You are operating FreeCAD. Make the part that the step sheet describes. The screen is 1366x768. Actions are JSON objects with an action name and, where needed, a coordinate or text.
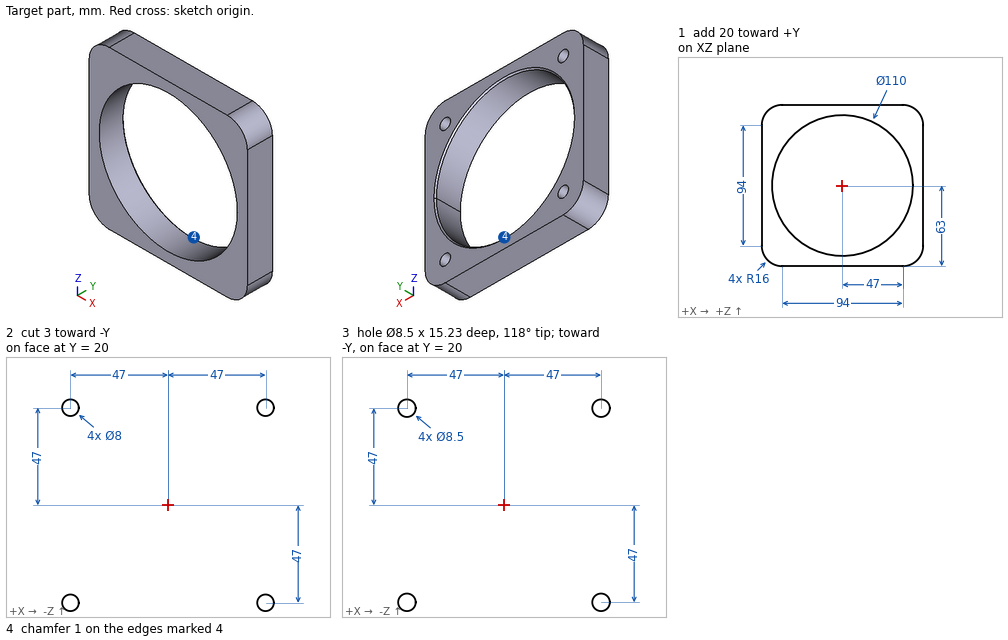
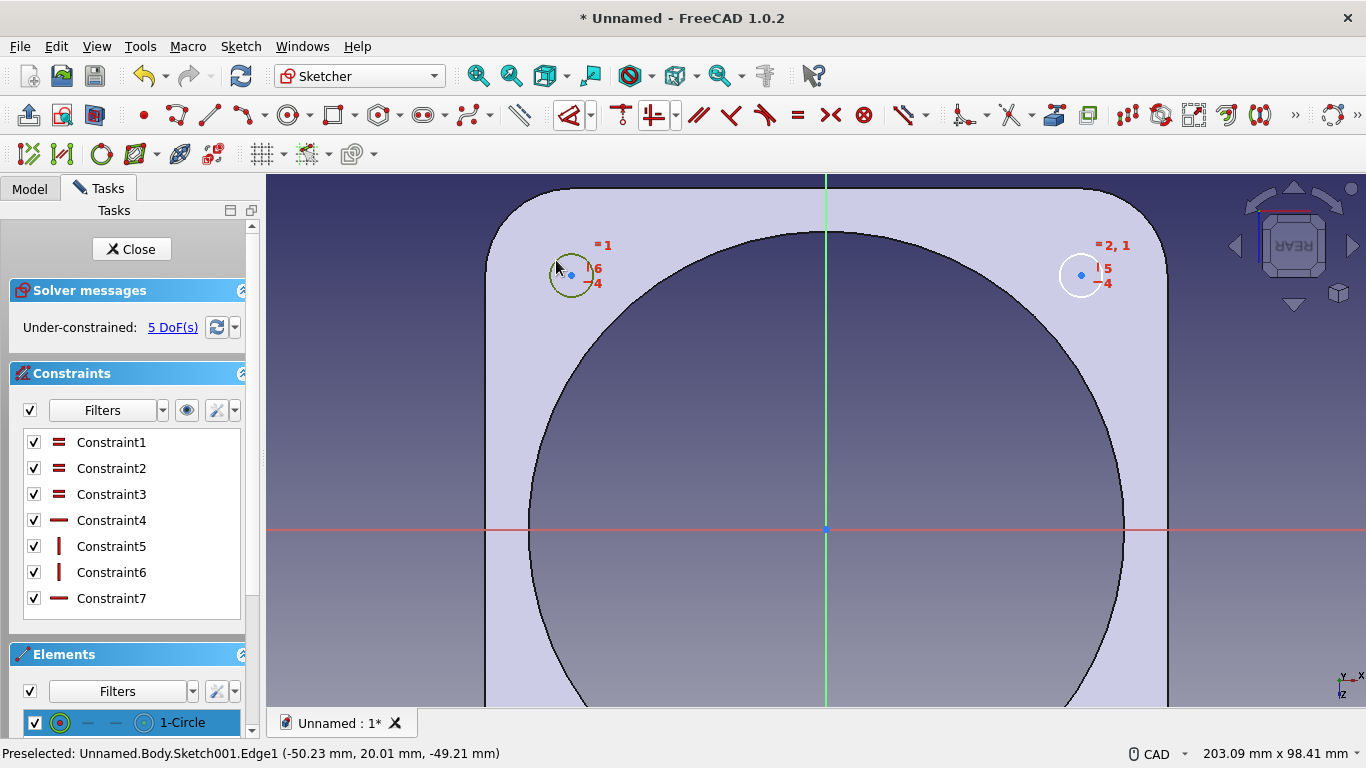
{"action": "left_click", "coordinate": [590, 116]}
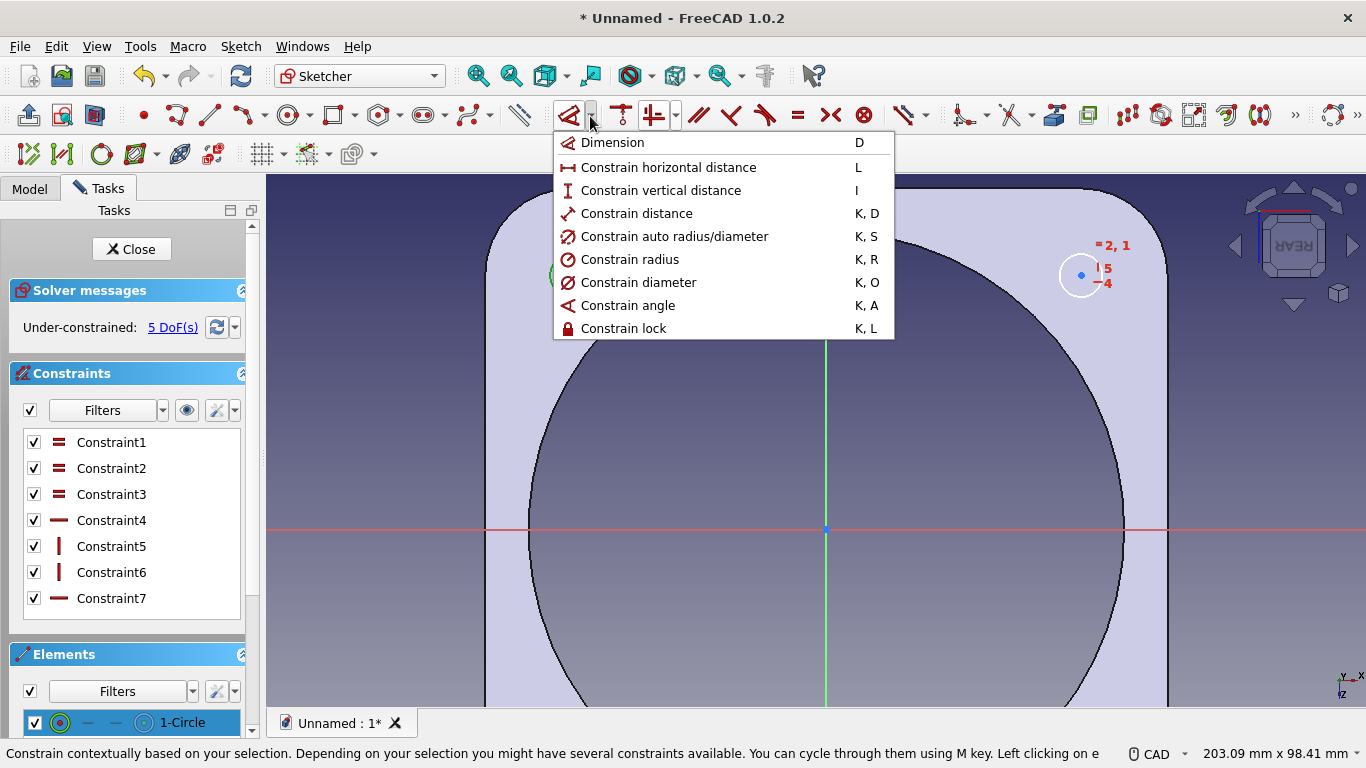
{"action": "left_click", "coordinate": [724, 282]}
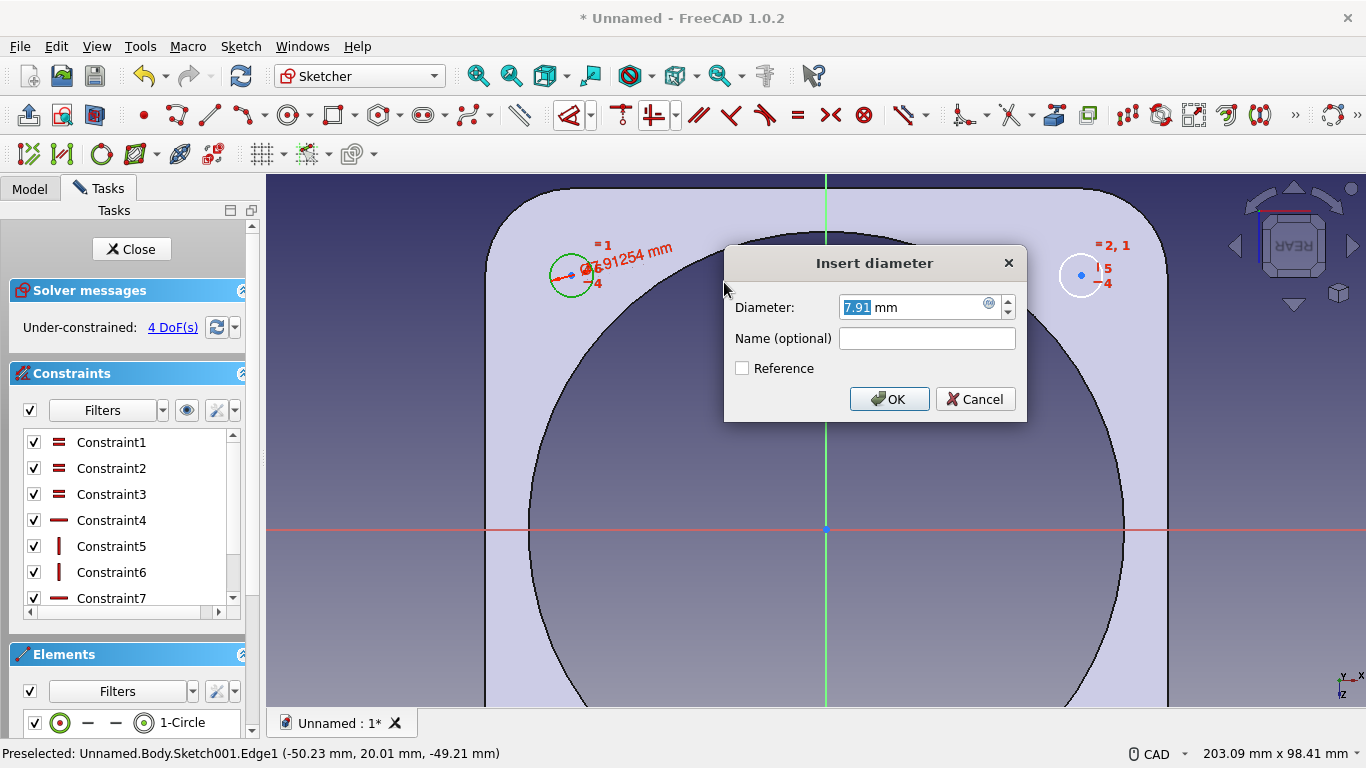
{"action": "type", "text": "8"}
{"action": "key", "text": "Return"}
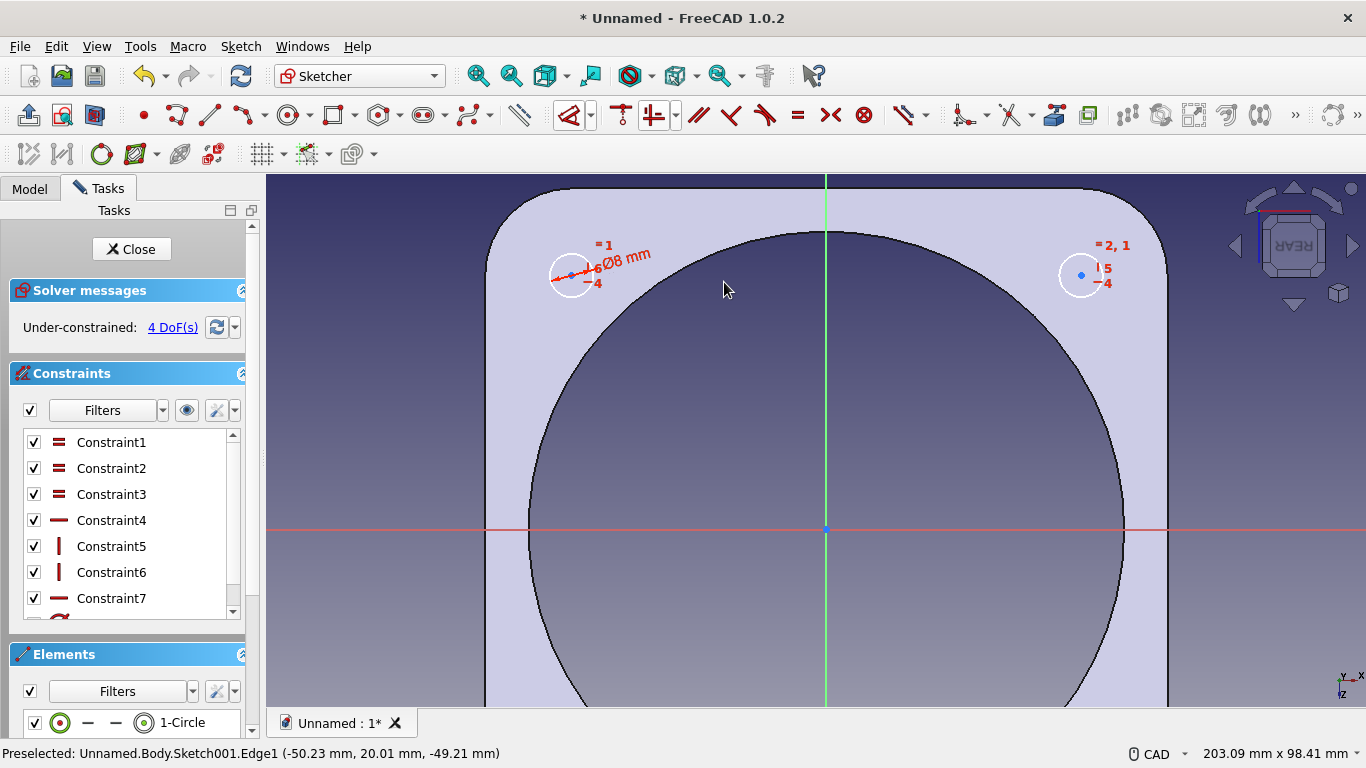
{"action": "left_click", "coordinate": [572, 276]}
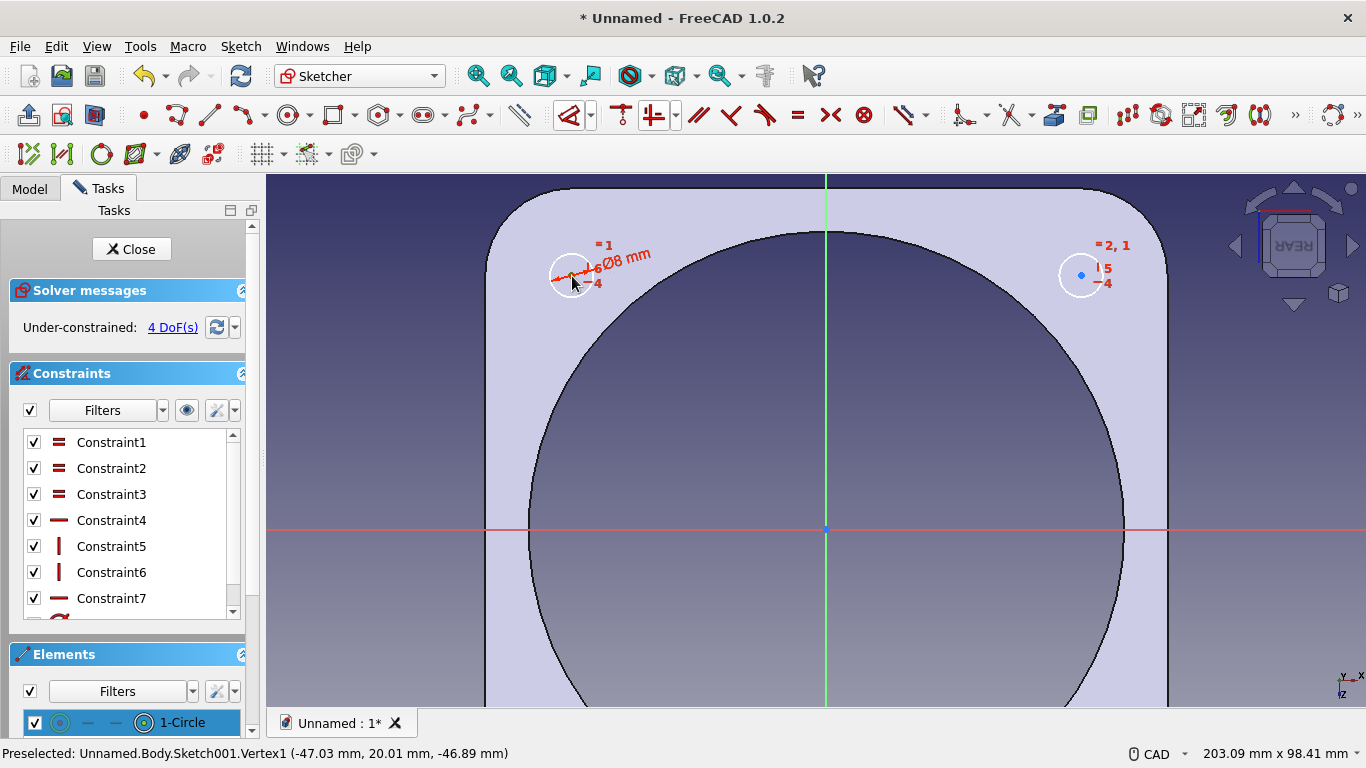
{"action": "key", "text": "l"}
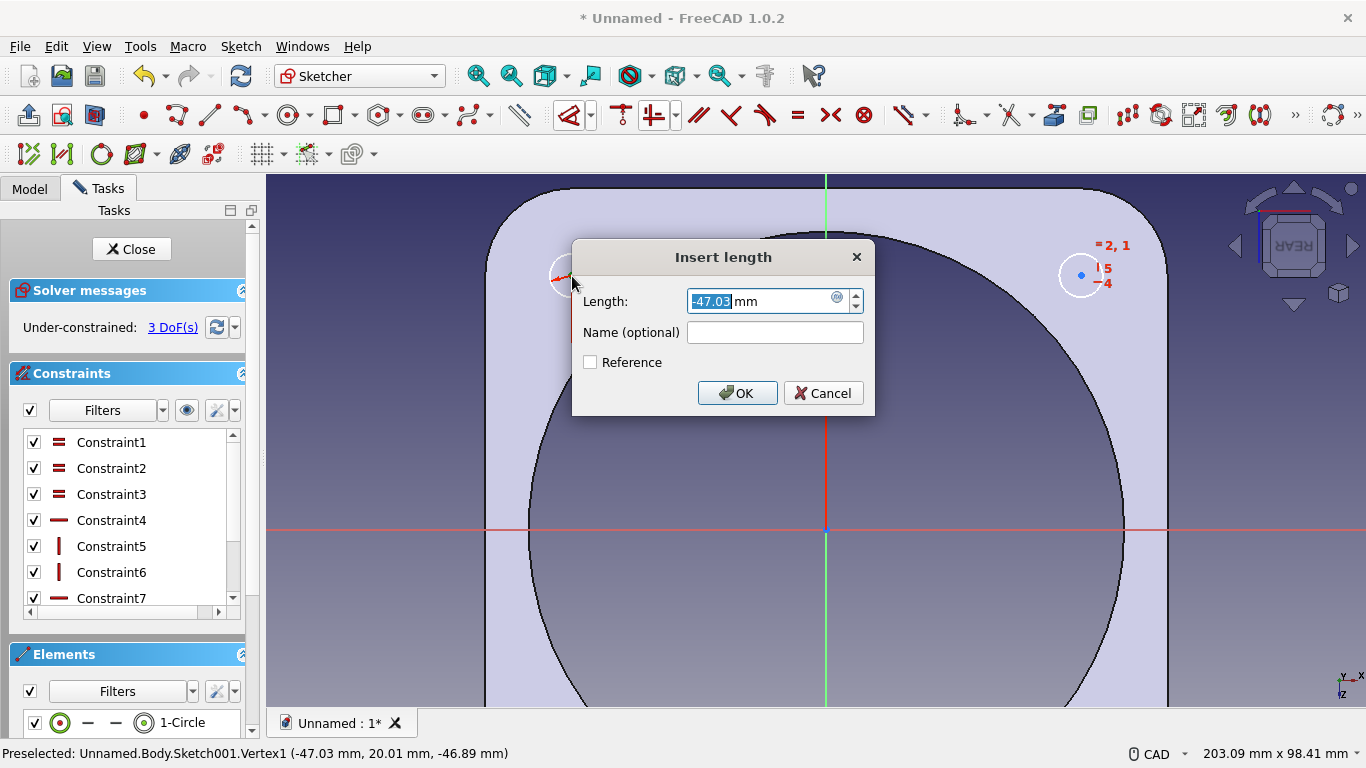
{"action": "type", "text": "-47"}
{"action": "key", "text": "Return"}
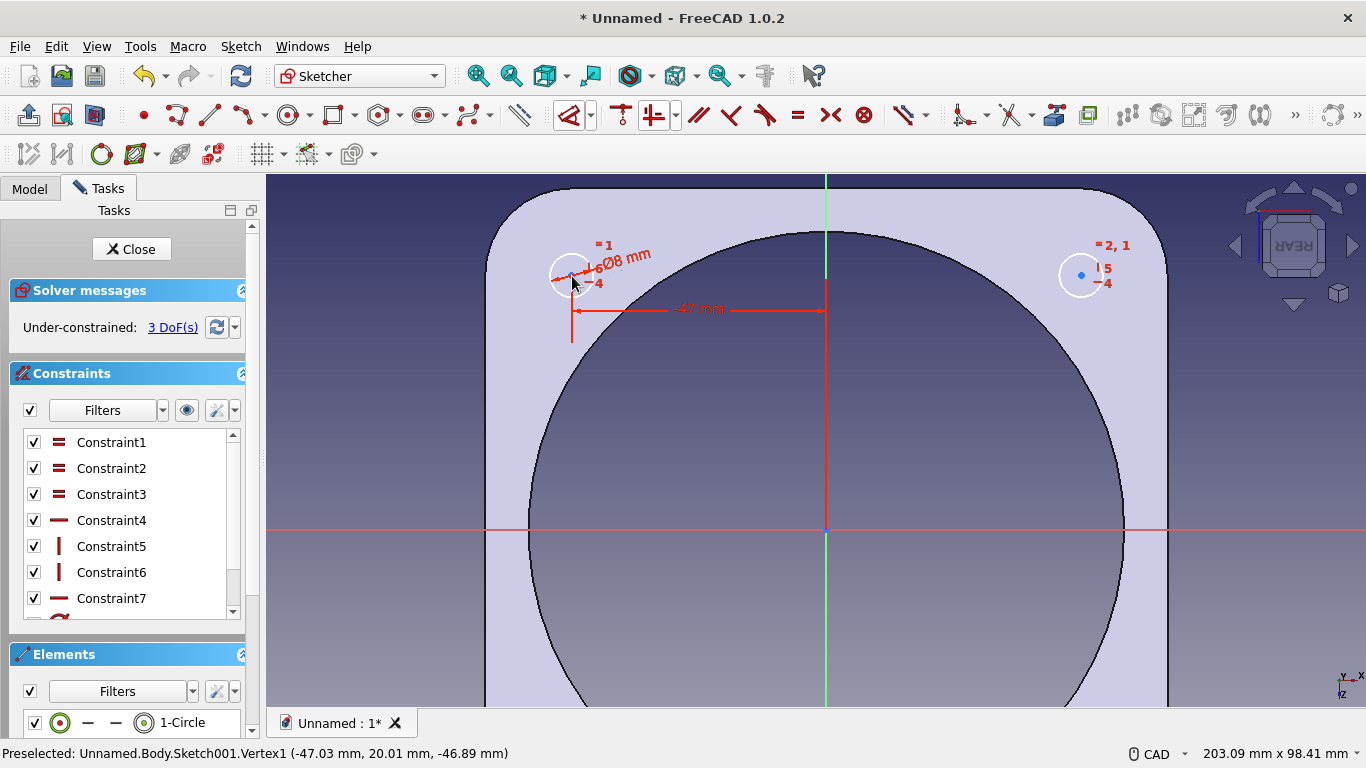
{"action": "left_click", "coordinate": [572, 276]}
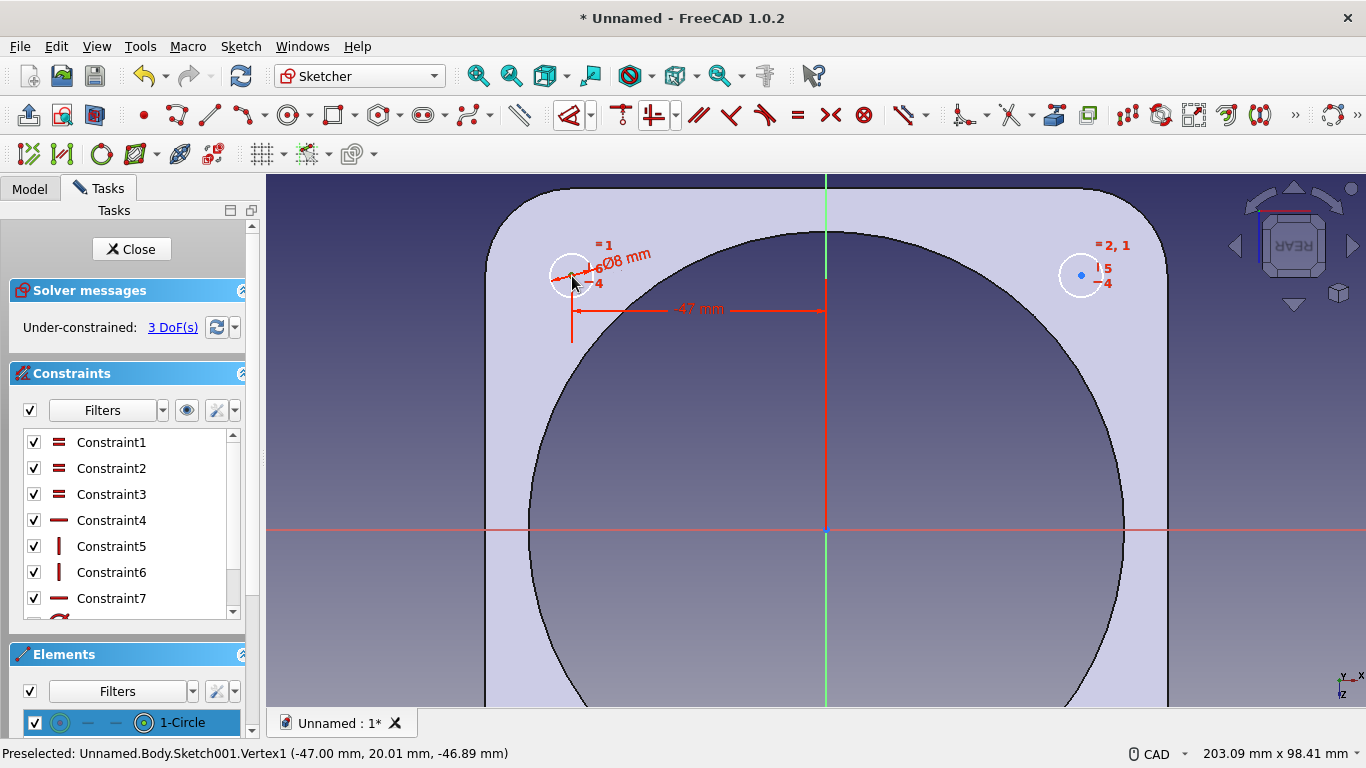
{"action": "left_click", "coordinate": [590, 116]}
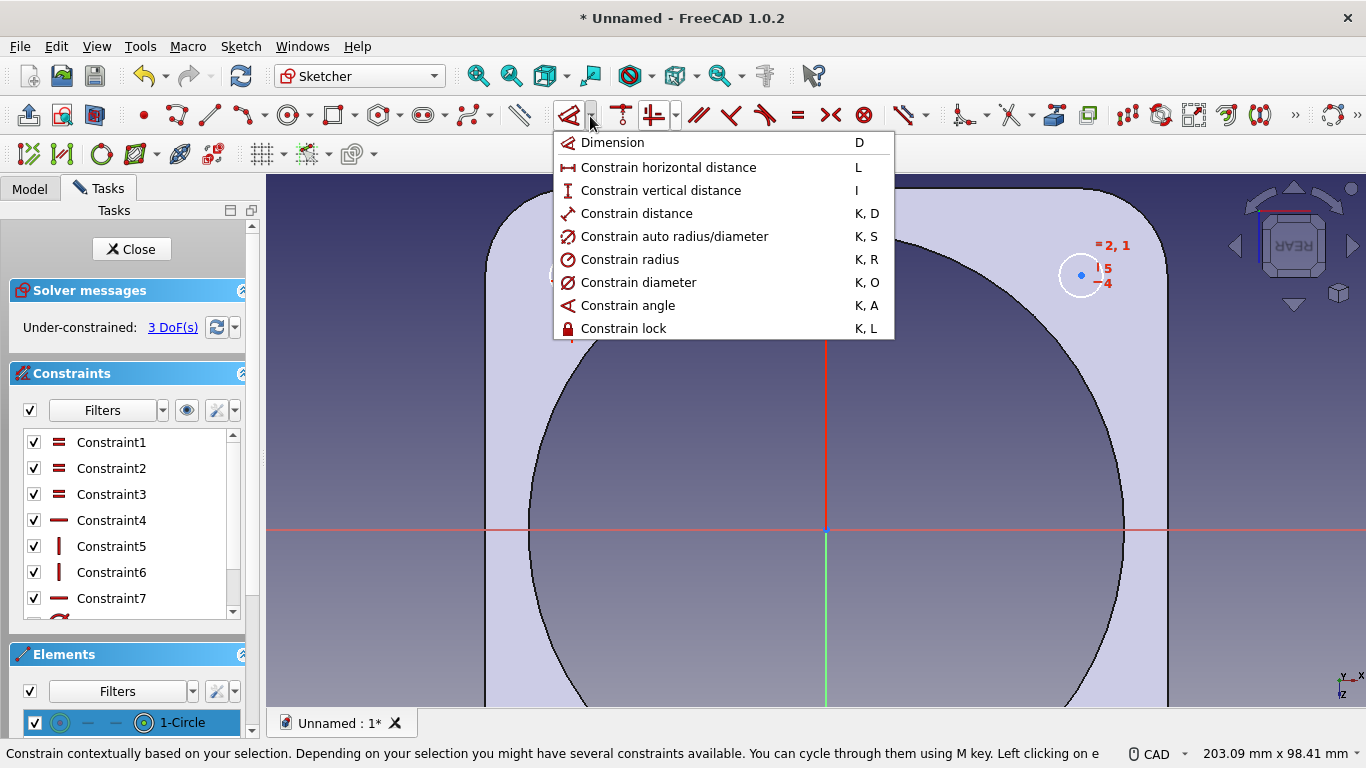
{"action": "left_click", "coordinate": [724, 190]}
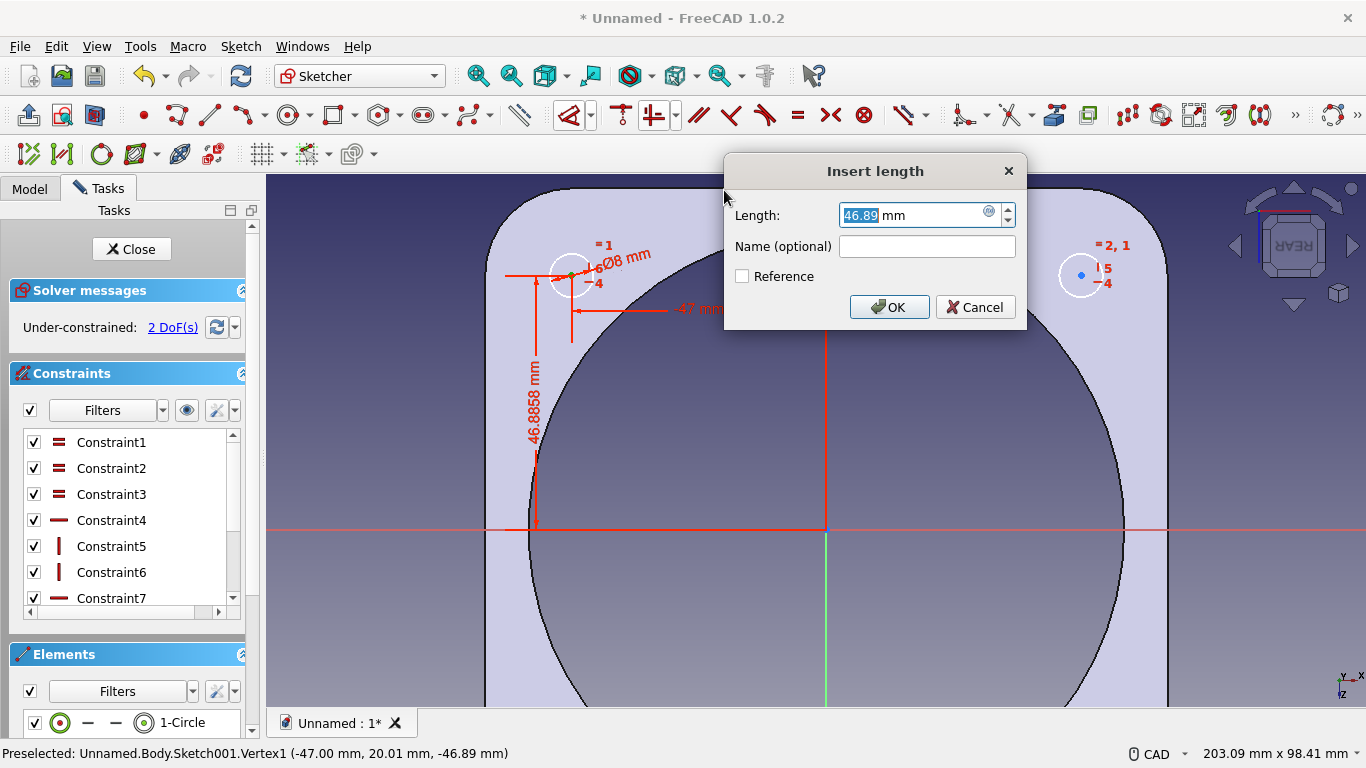
{"action": "type", "text": "47"}
{"action": "key", "text": "Return"}